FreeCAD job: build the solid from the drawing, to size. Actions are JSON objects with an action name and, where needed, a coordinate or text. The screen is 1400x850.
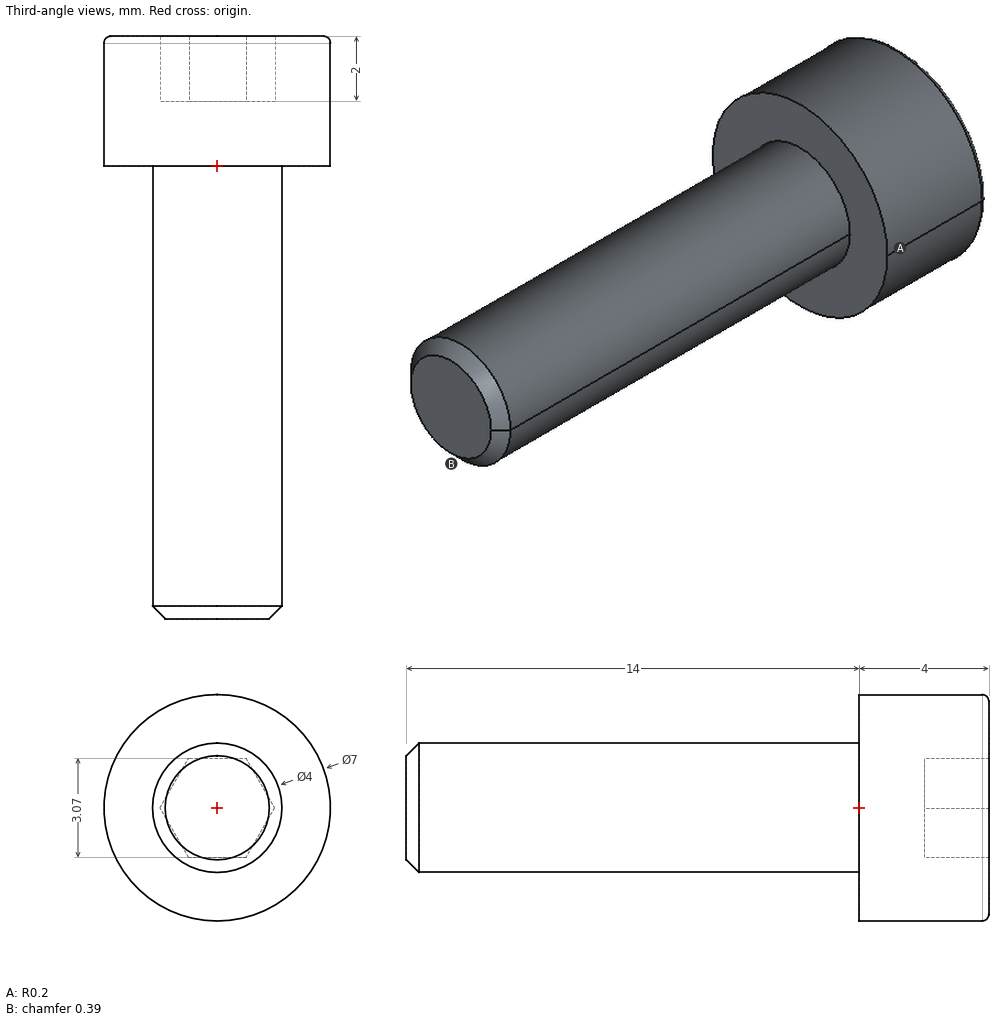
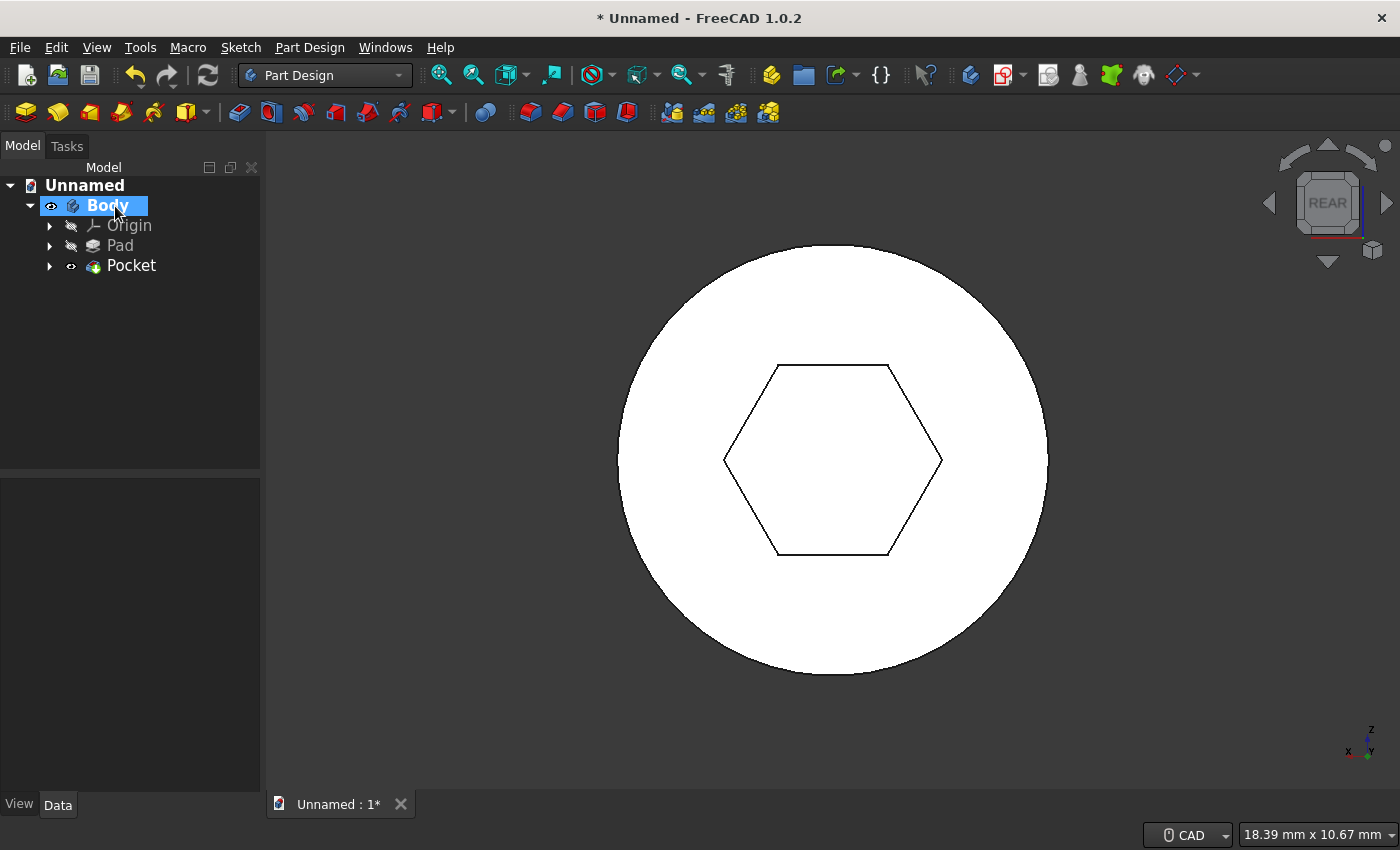
{"action": "left_click", "coordinate": [1049, 459]}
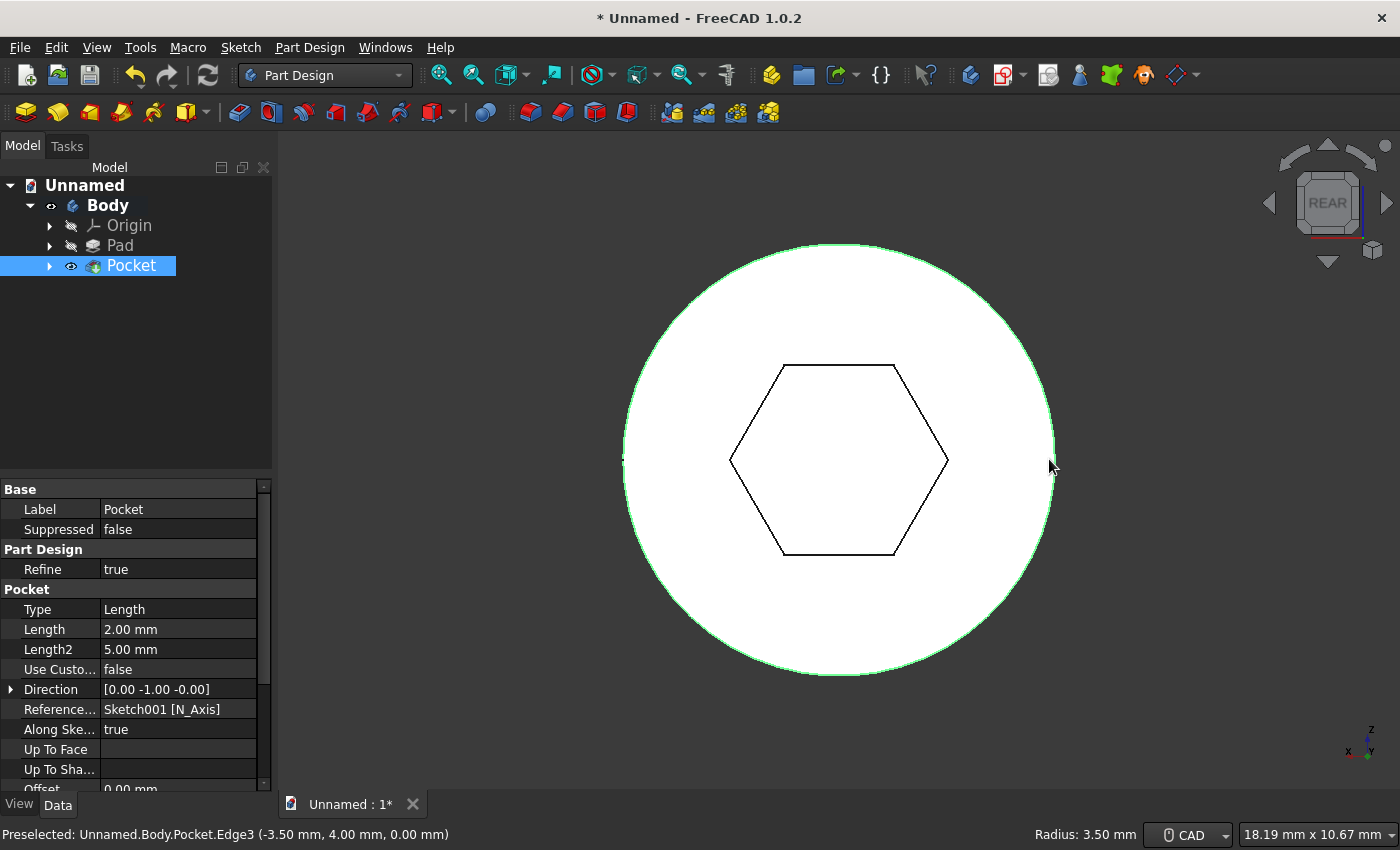
{"action": "left_click", "coordinate": [532, 112]}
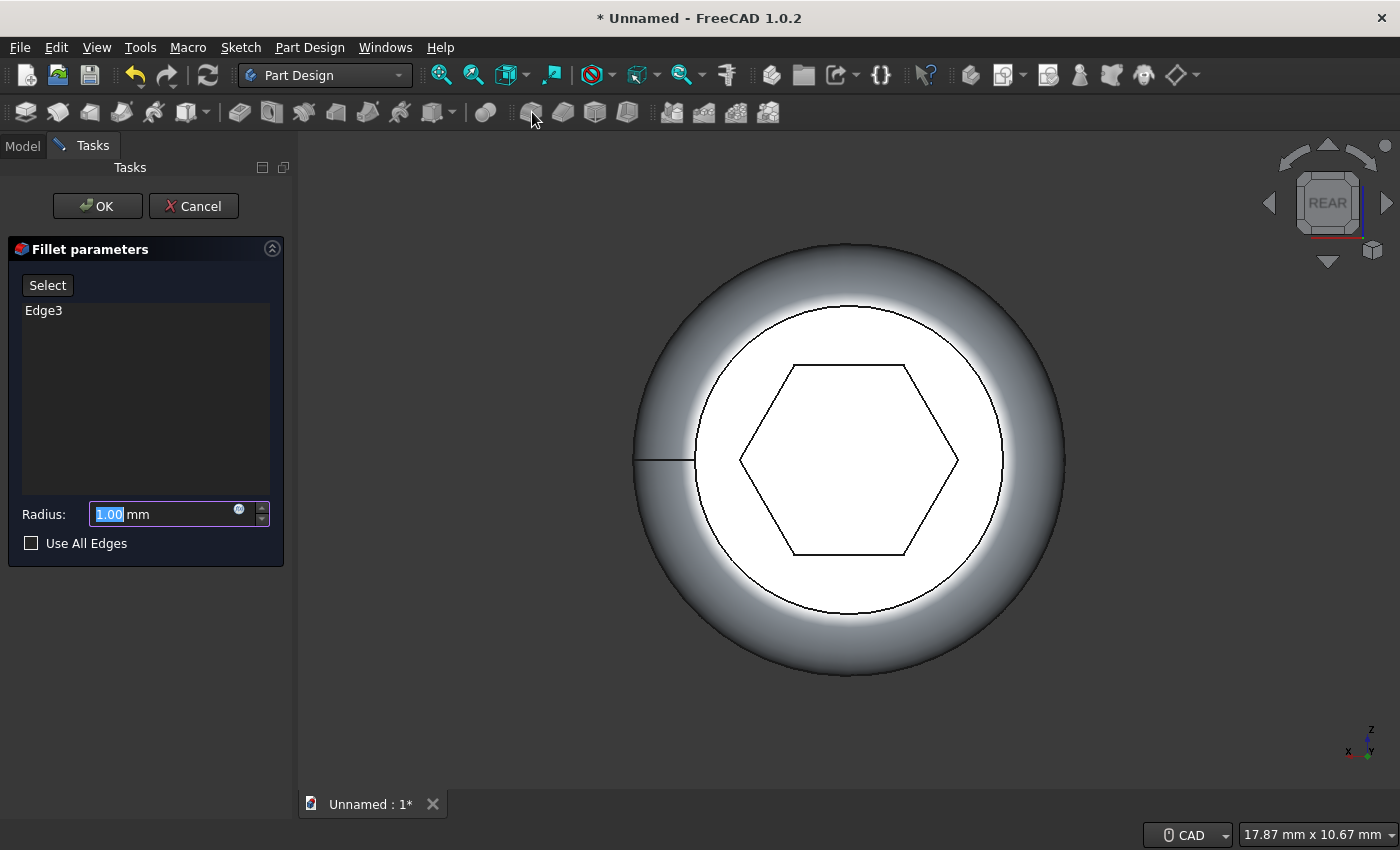
{"action": "type", "text": "0.2"}
{"action": "key", "text": "Tab"}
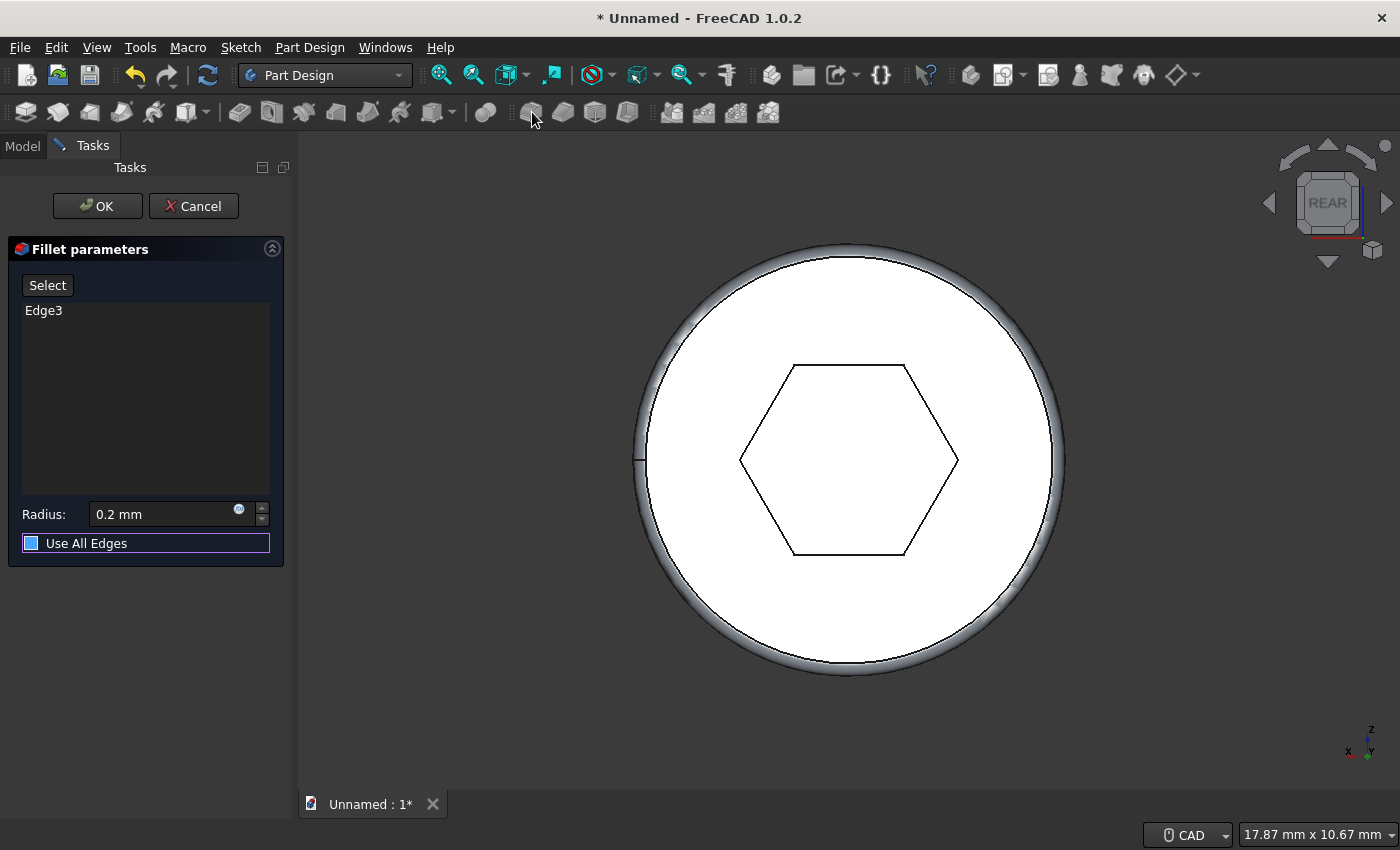
{"action": "left_click", "coordinate": [98, 206]}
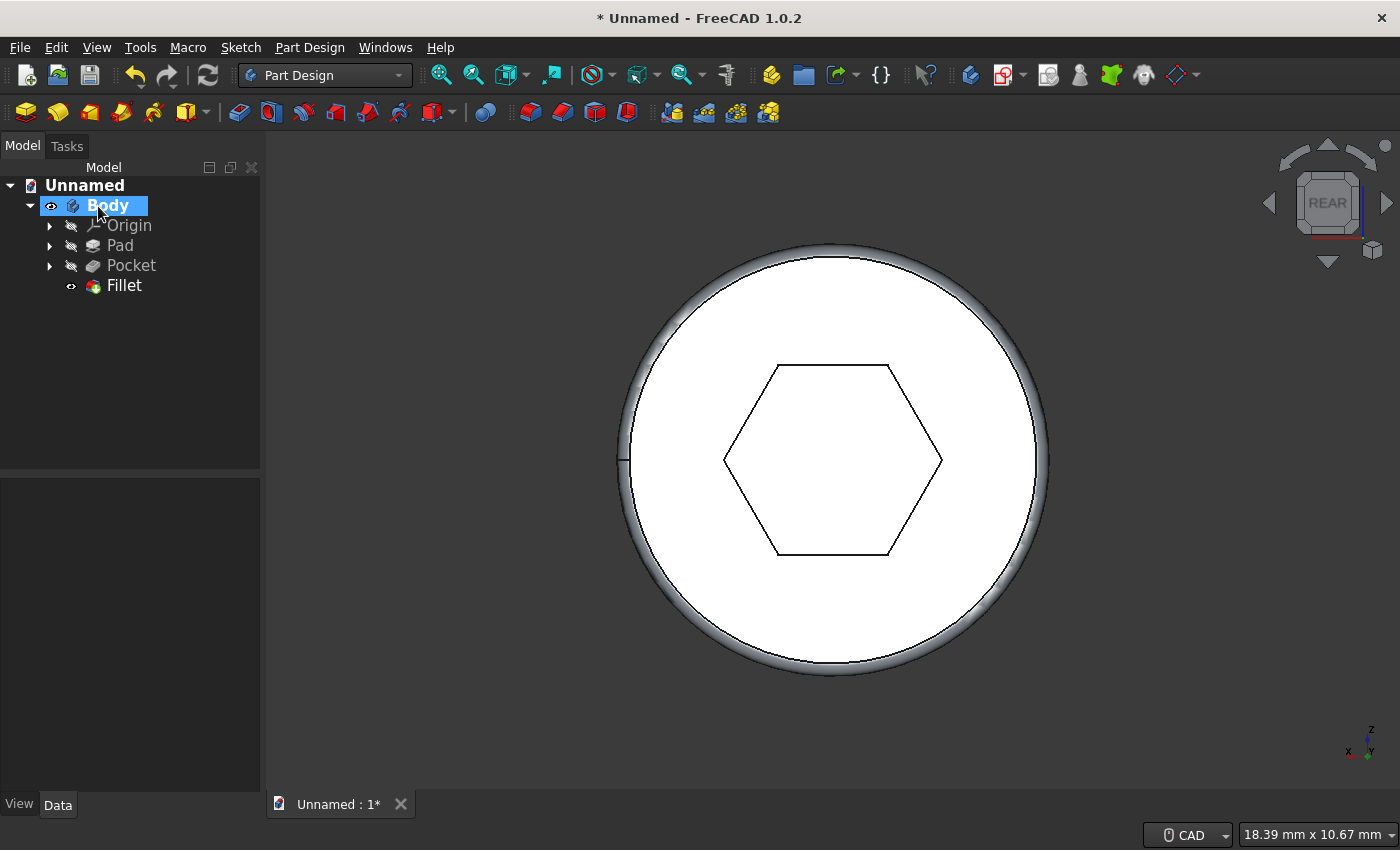
{"action": "left_click", "coordinate": [1004, 76]}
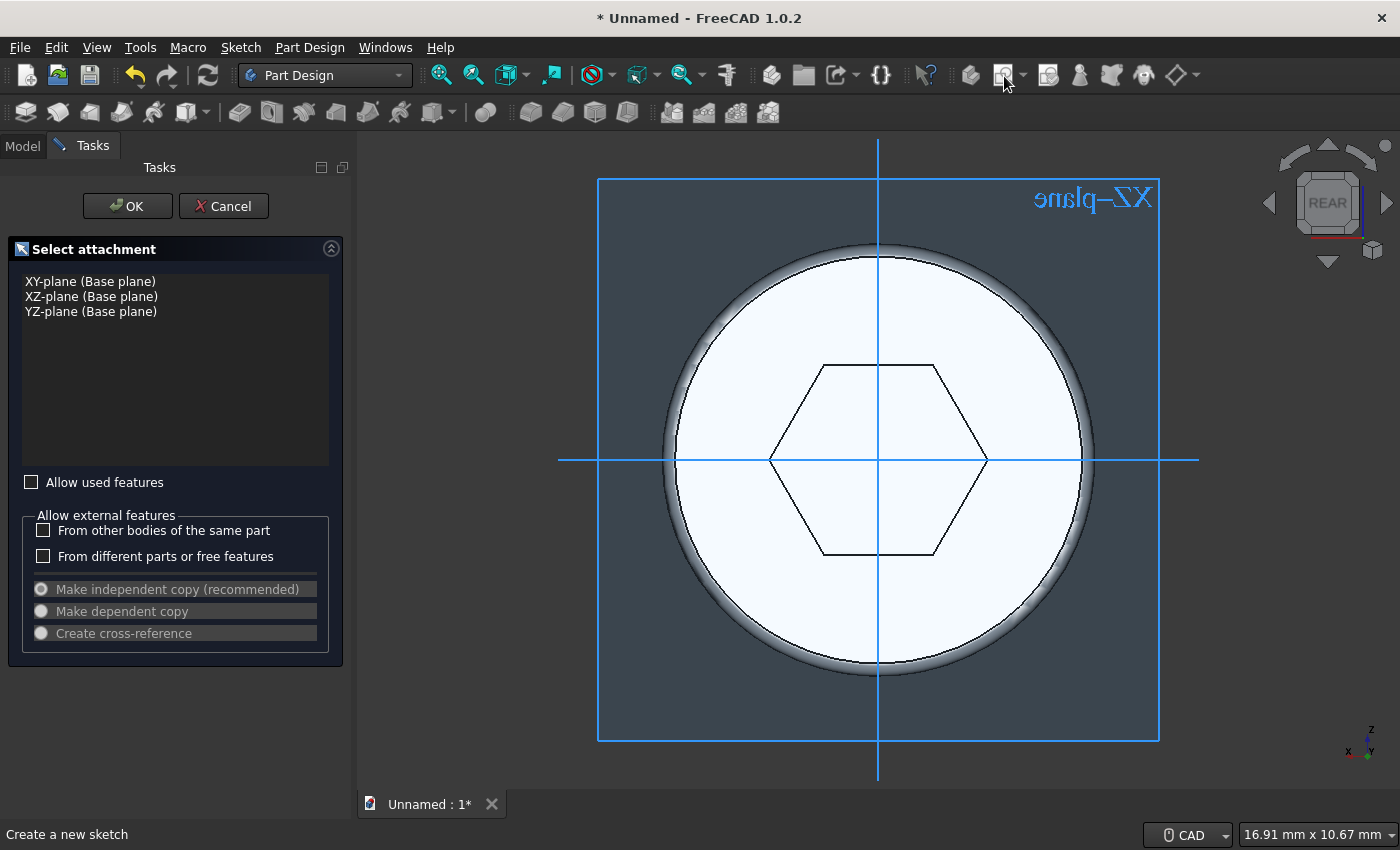
{"action": "left_click", "coordinate": [82, 296]}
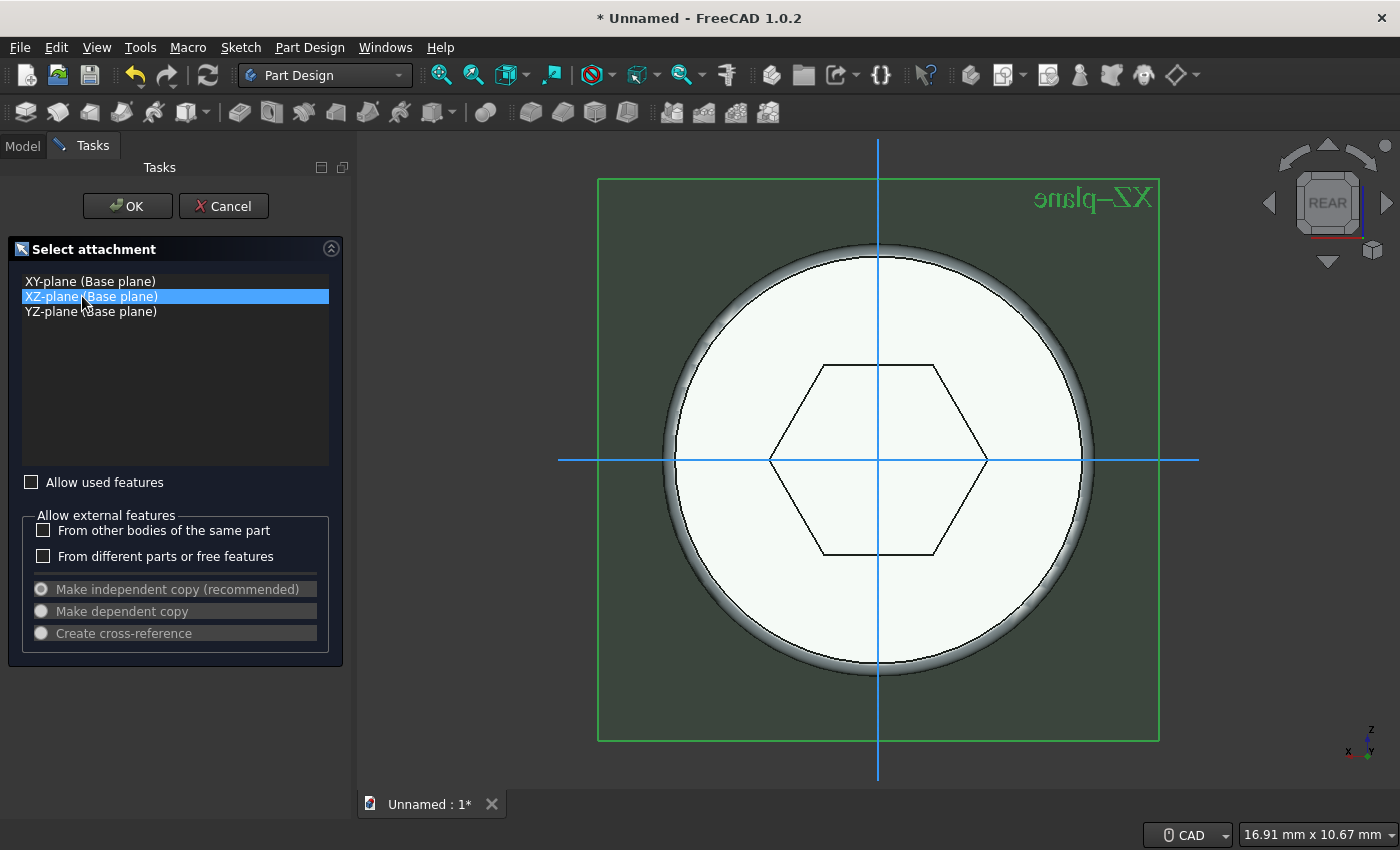
{"action": "left_click", "coordinate": [128, 206]}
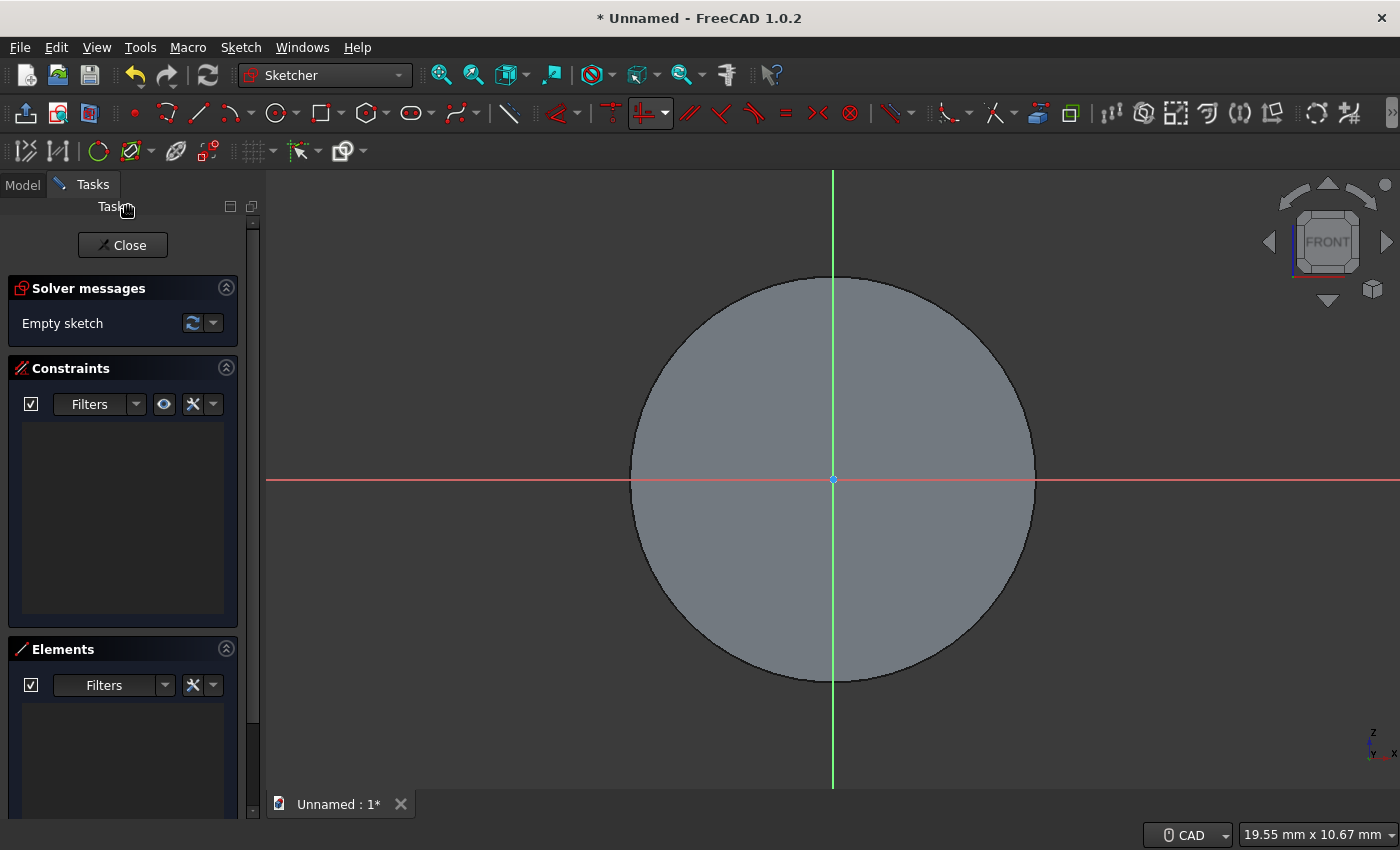
{"action": "scroll", "coordinate": [916, 480], "scroll_direction": "up", "scroll_amount": 3}